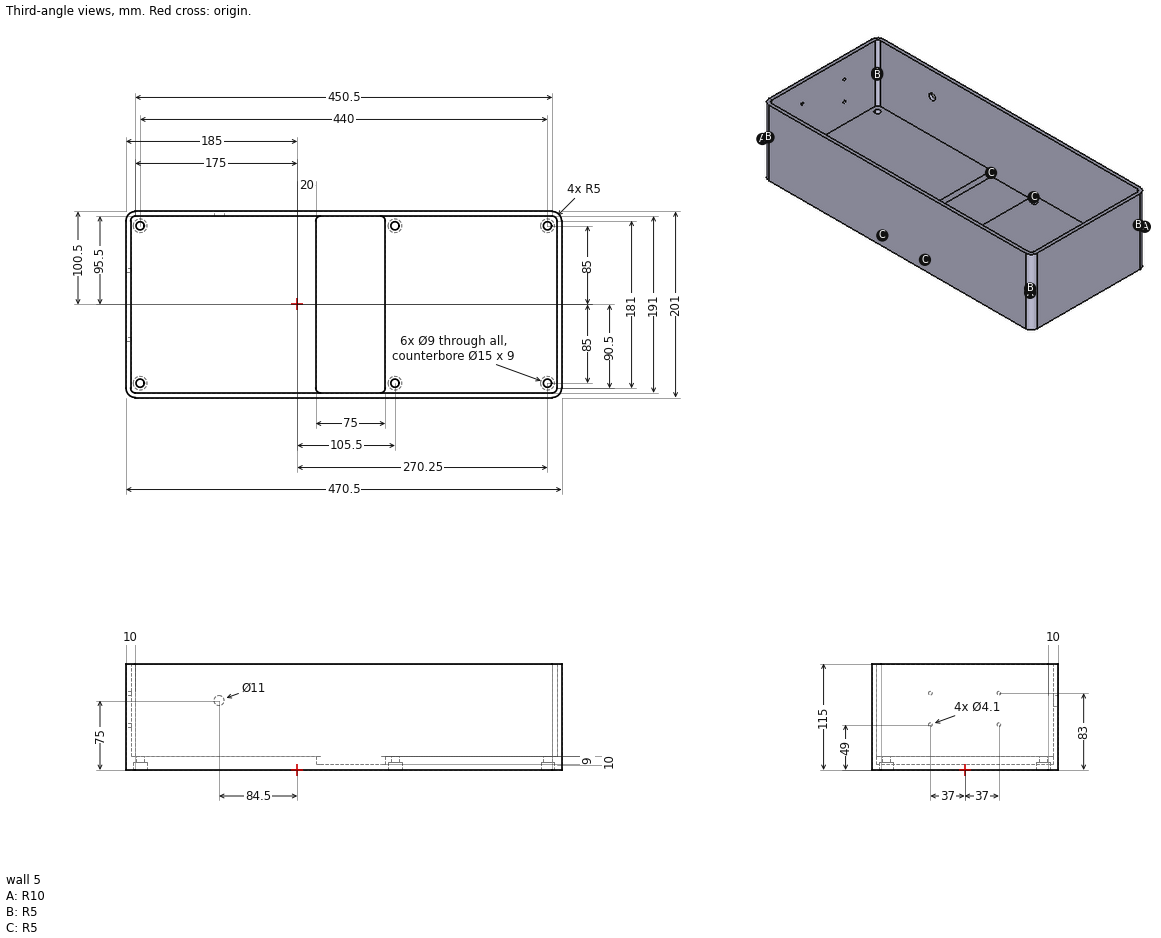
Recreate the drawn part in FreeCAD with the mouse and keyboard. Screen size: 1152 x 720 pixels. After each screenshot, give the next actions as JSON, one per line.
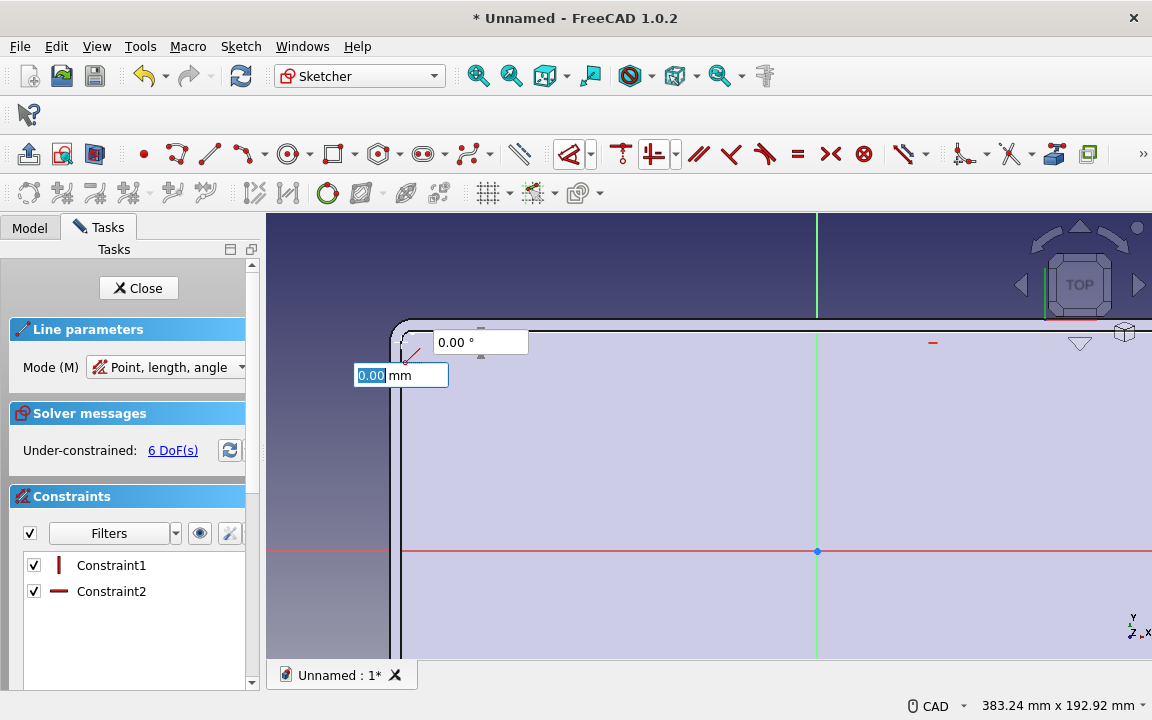
{"action": "scroll", "coordinate": [401, 342], "scroll_direction": "down", "scroll_amount": 4}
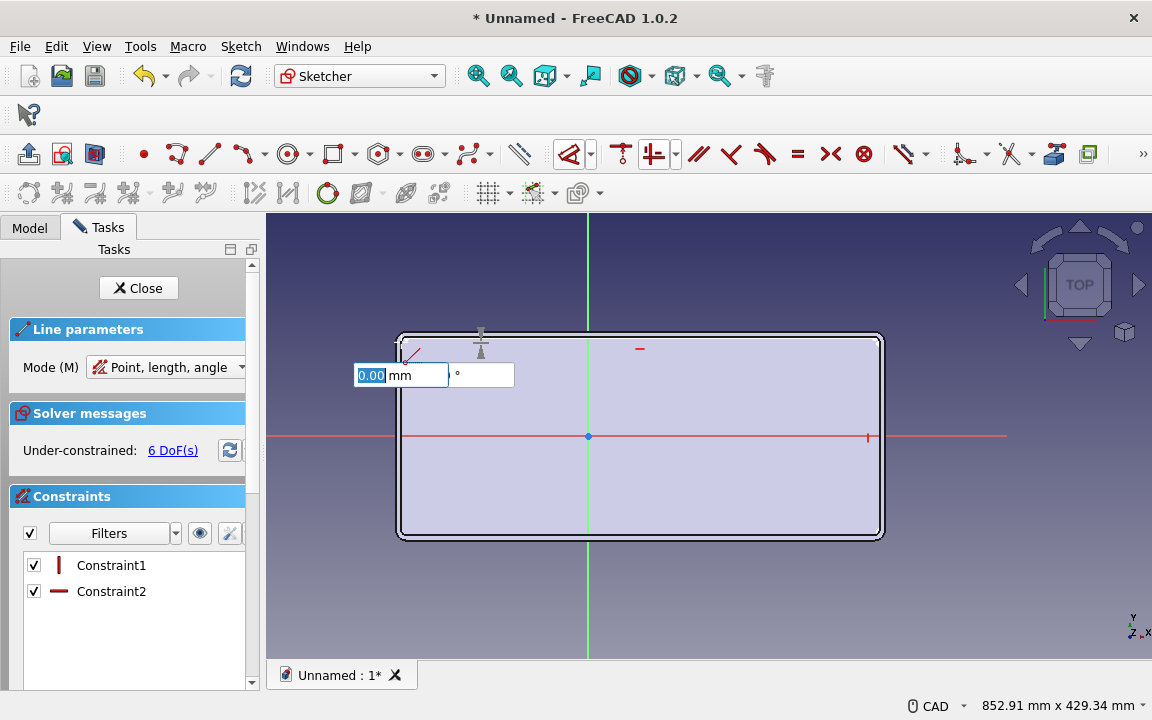
{"action": "left_click", "coordinate": [401, 530]}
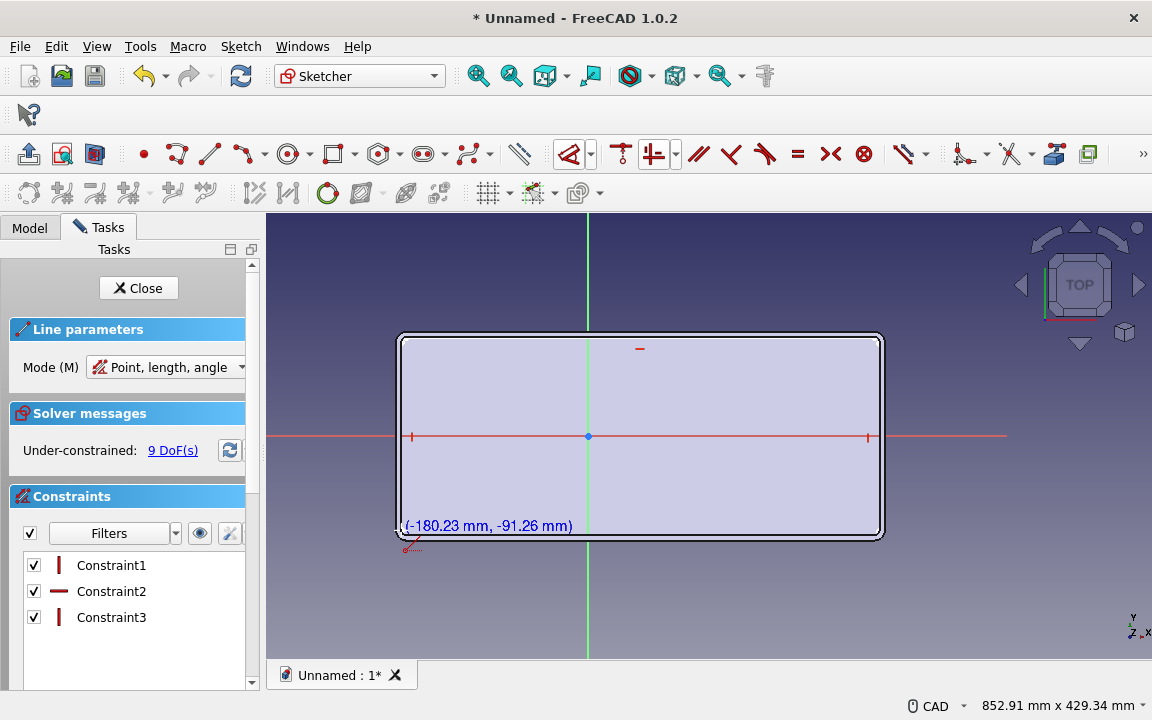
{"action": "scroll", "coordinate": [406, 535], "scroll_direction": "up", "scroll_amount": 4}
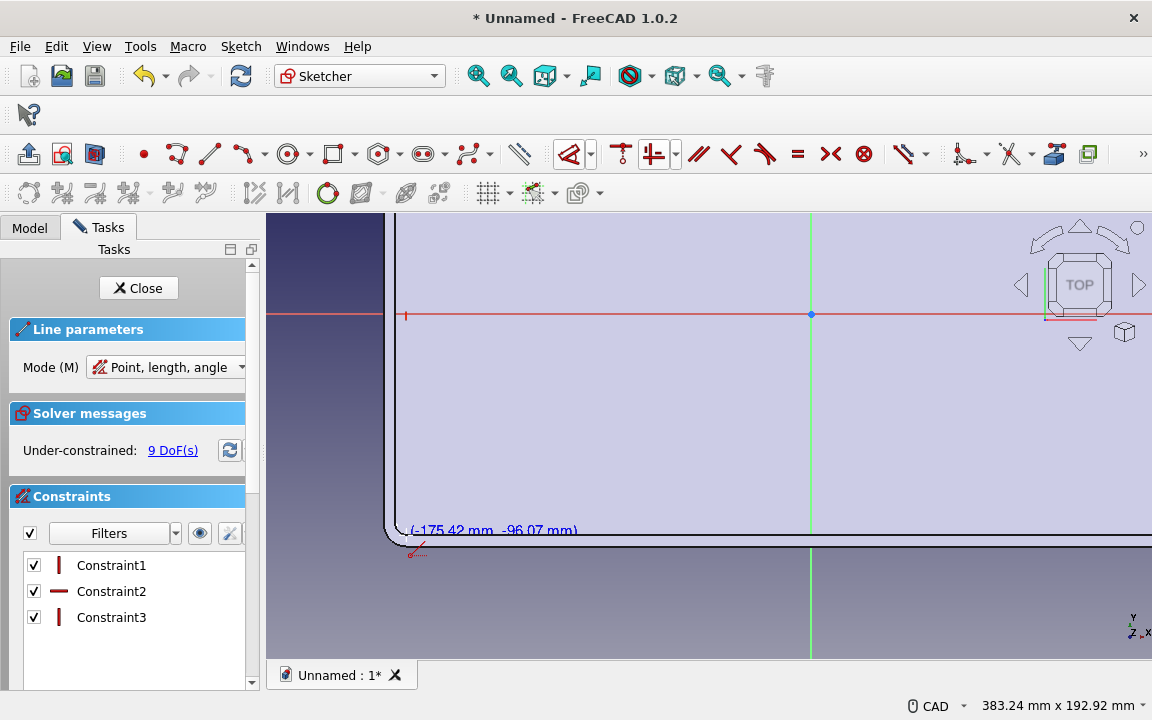
{"action": "left_click", "coordinate": [407, 535]}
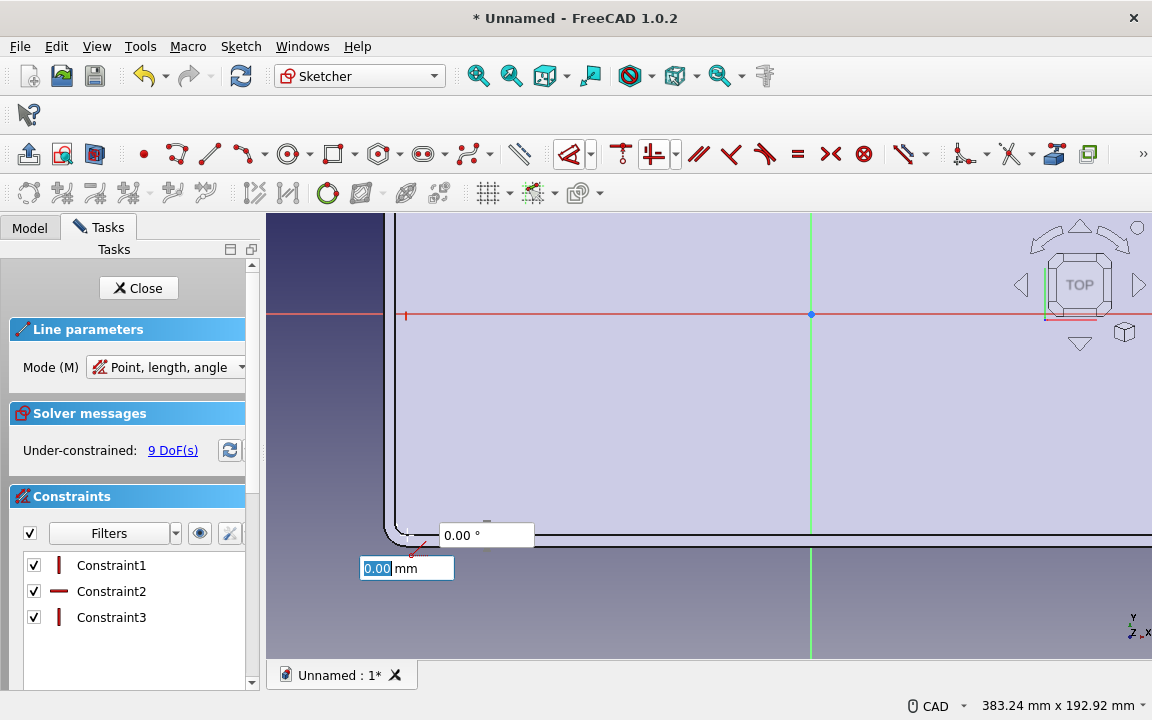
{"action": "scroll", "coordinate": [406, 535], "scroll_direction": "down", "scroll_amount": 4}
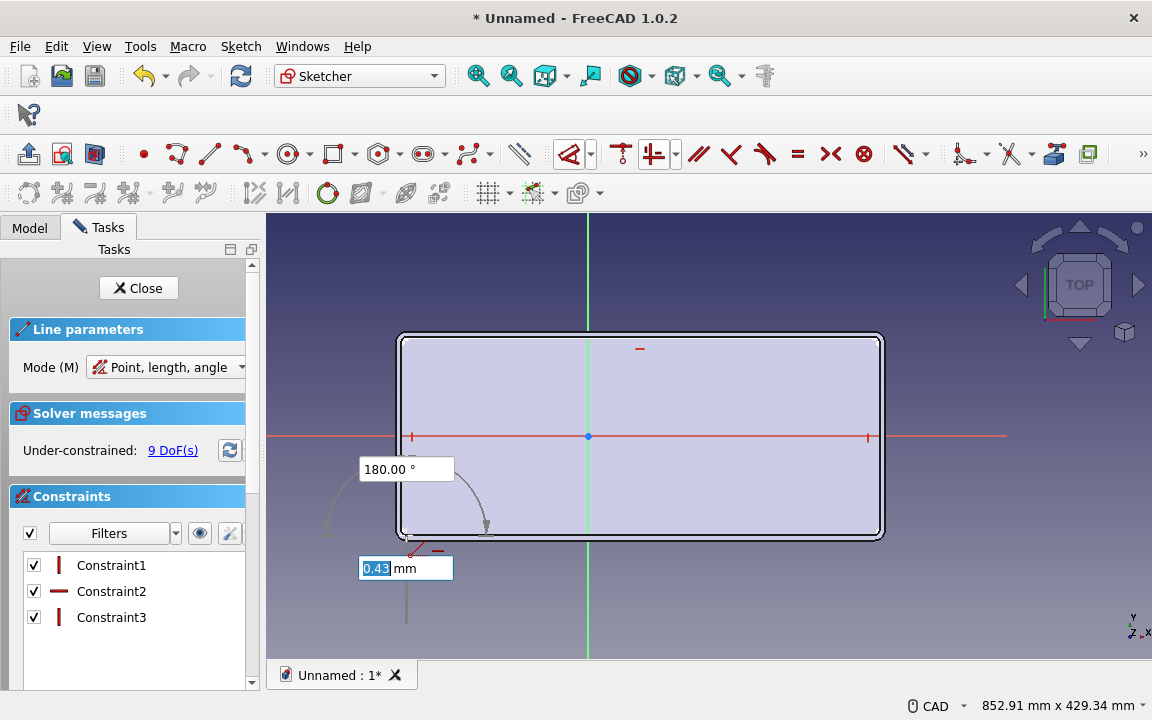
{"action": "scroll", "coordinate": [874, 535], "scroll_direction": "up", "scroll_amount": 4}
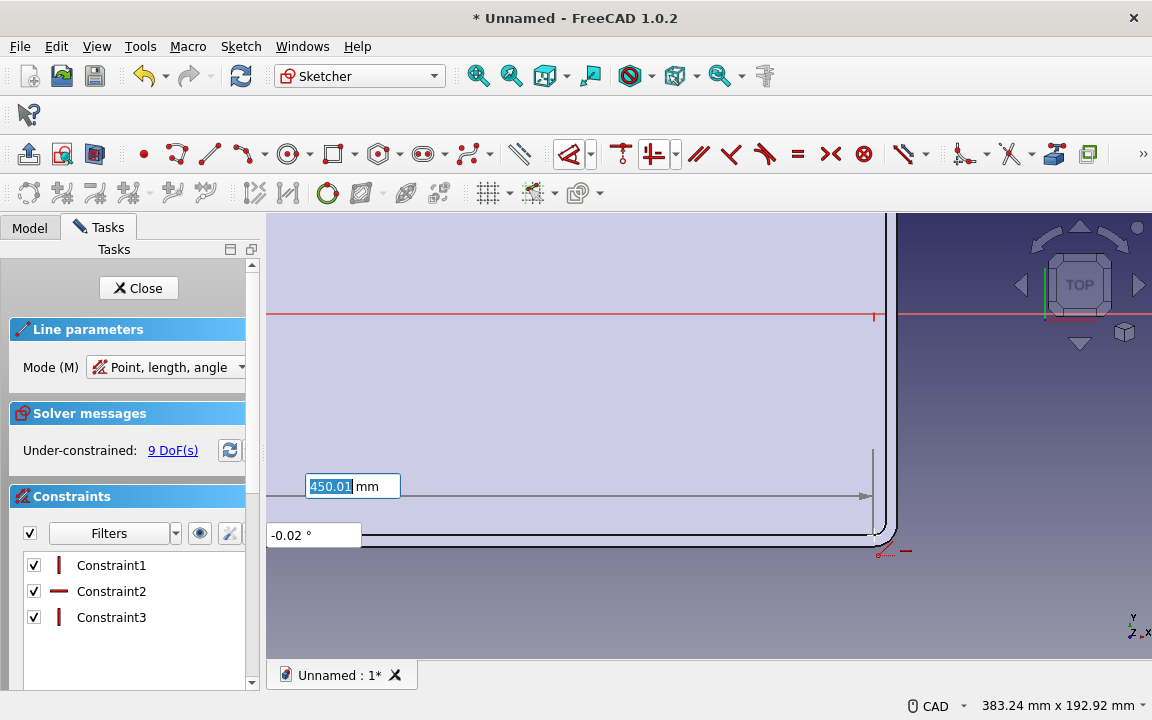
{"action": "left_click", "coordinate": [874, 535]}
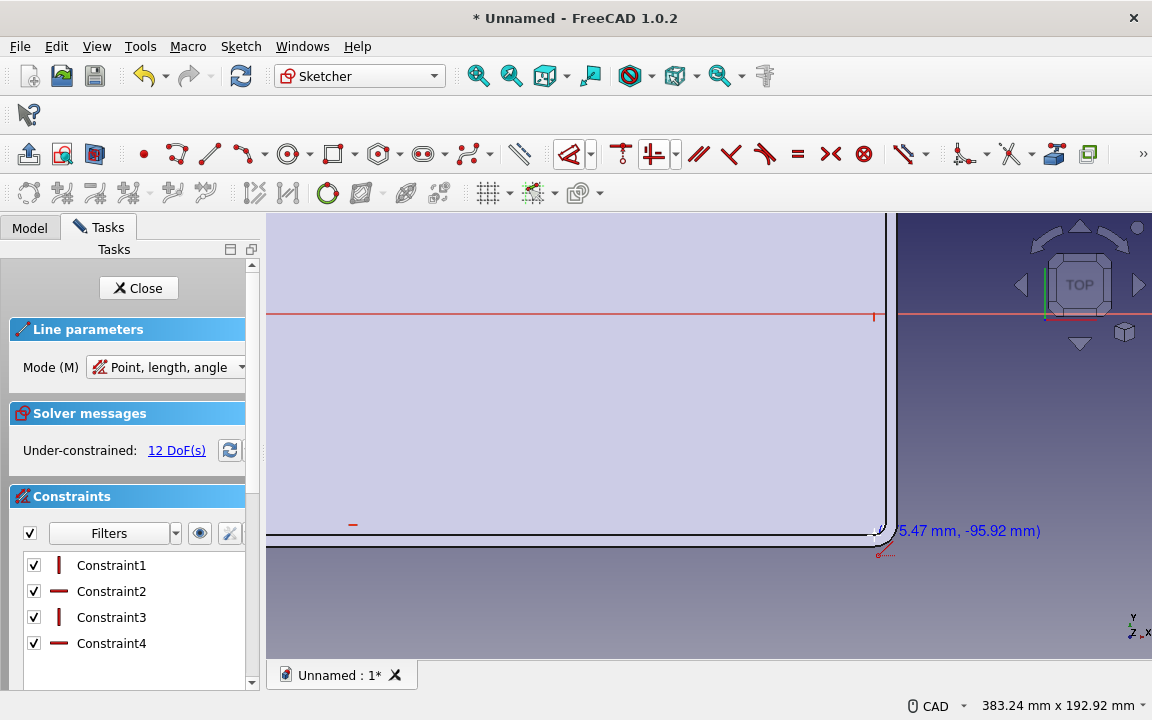
{"action": "key", "text": "g 3 a"}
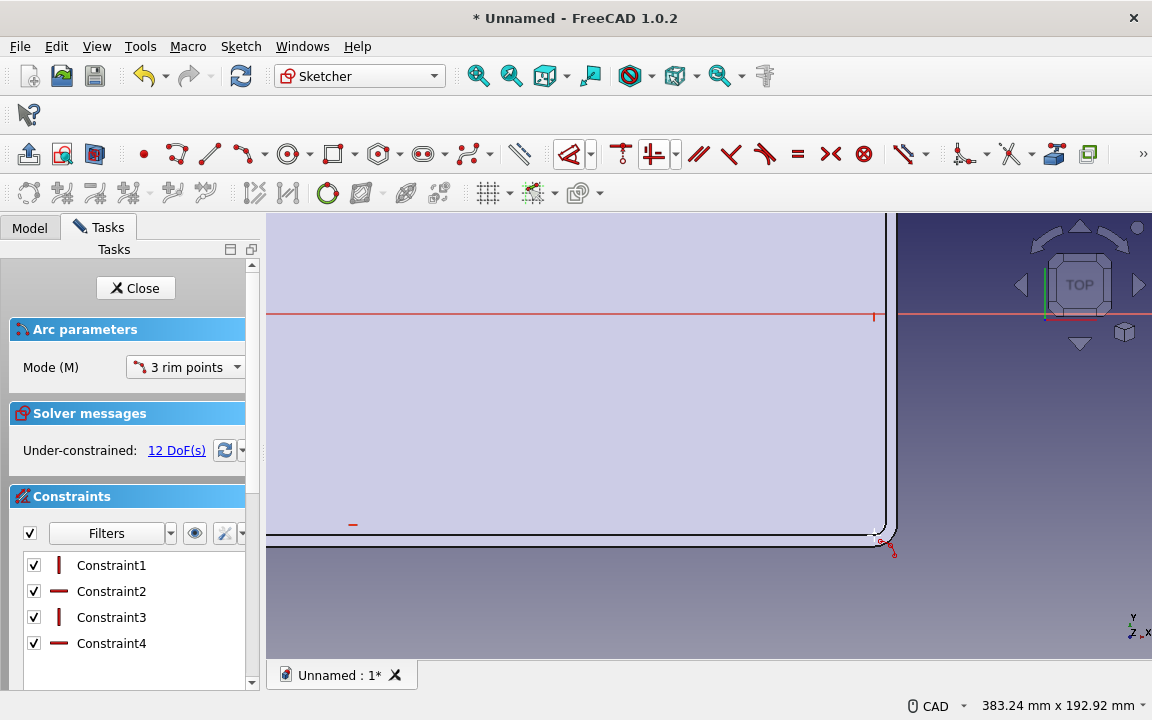
{"action": "scroll", "coordinate": [875, 535], "scroll_direction": "down", "scroll_amount": 4}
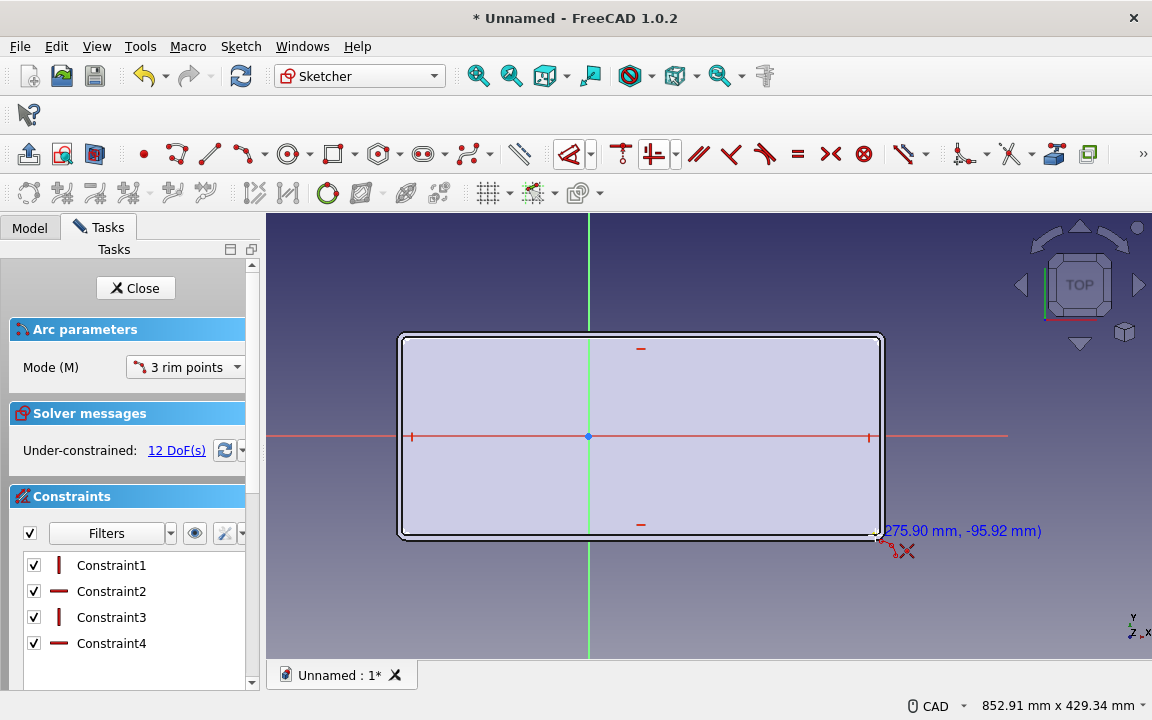
{"action": "scroll", "coordinate": [880, 342], "scroll_direction": "up", "scroll_amount": 4}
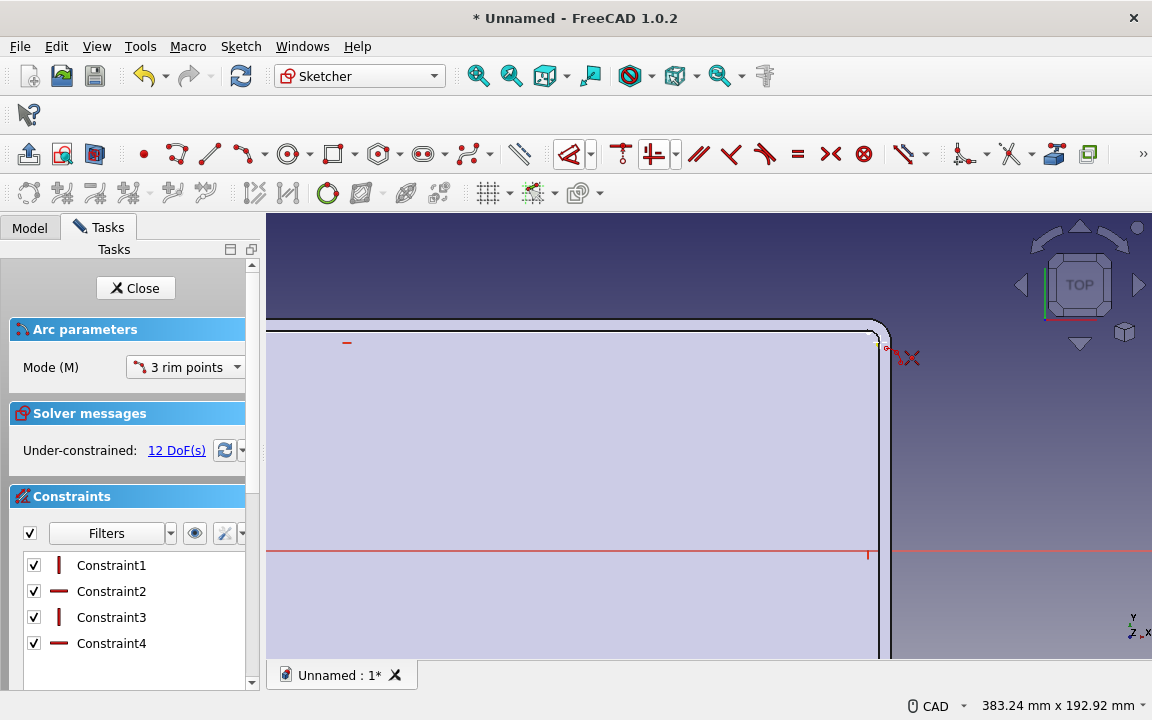
{"action": "left_click", "coordinate": [880, 345]}
{"action": "left_click", "coordinate": [868, 332]}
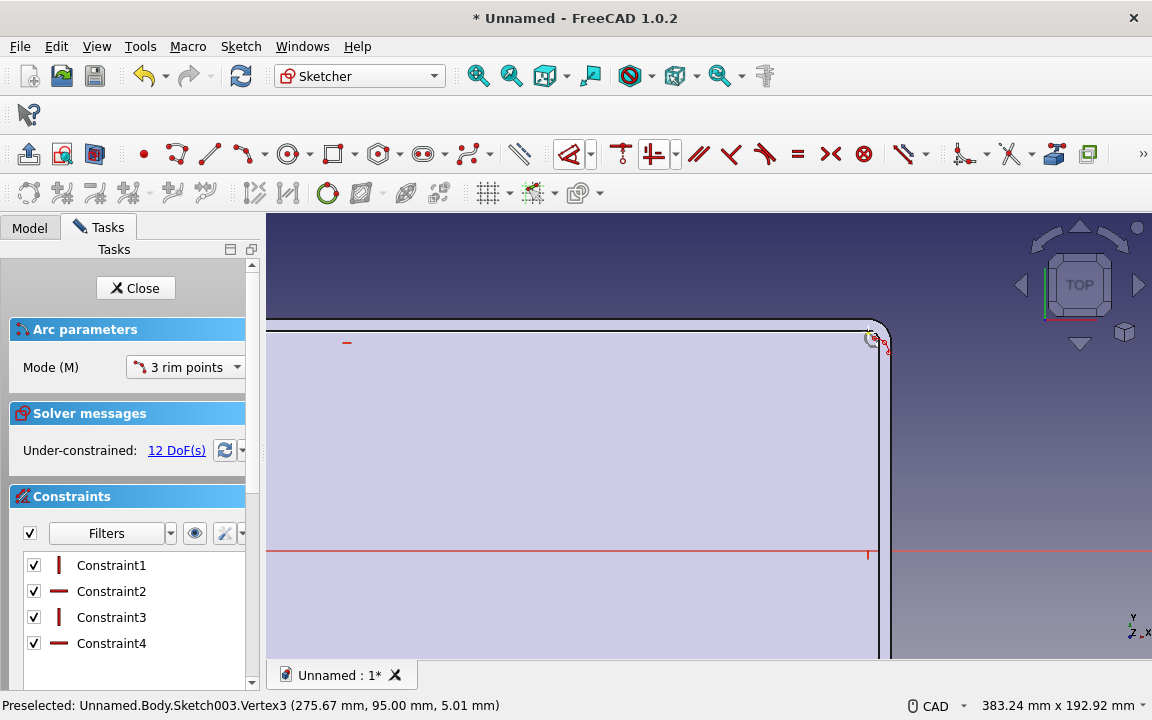
{"action": "scroll", "coordinate": [876, 334], "scroll_direction": "up", "scroll_amount": 8}